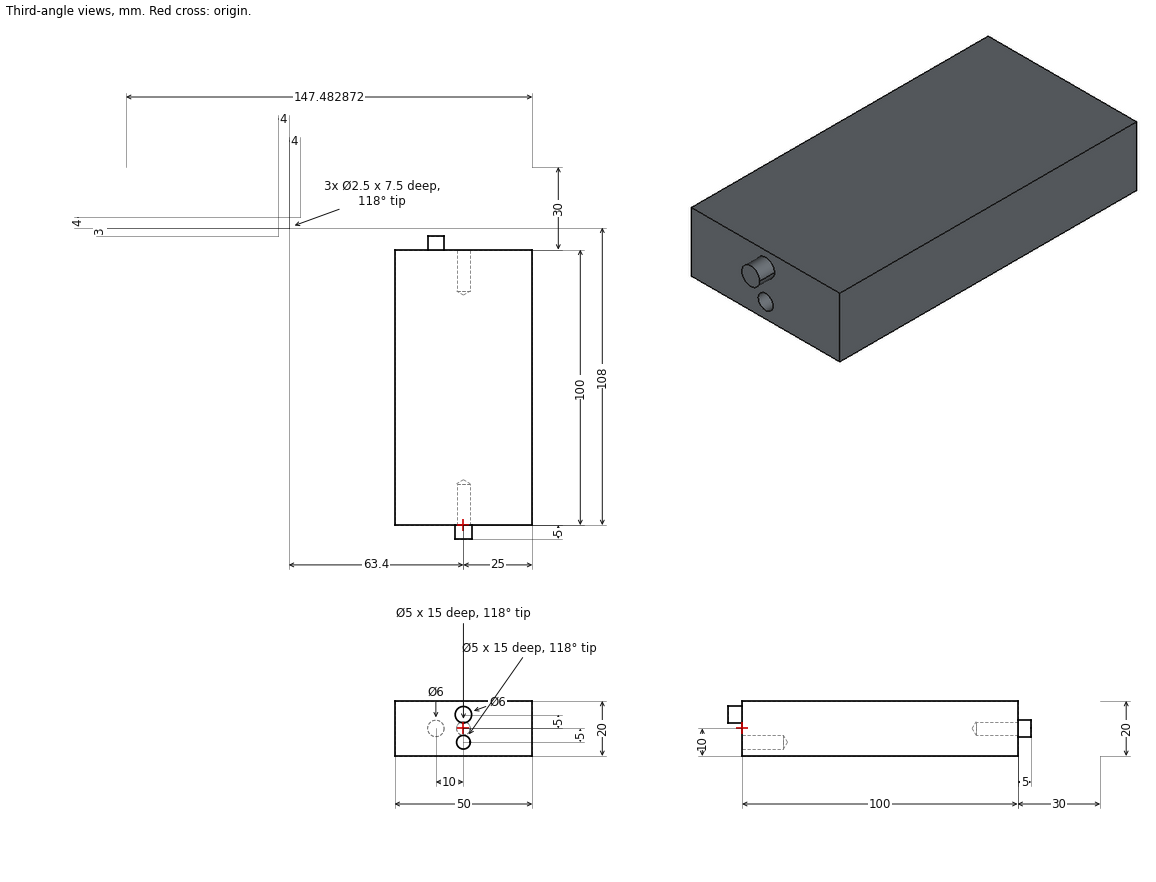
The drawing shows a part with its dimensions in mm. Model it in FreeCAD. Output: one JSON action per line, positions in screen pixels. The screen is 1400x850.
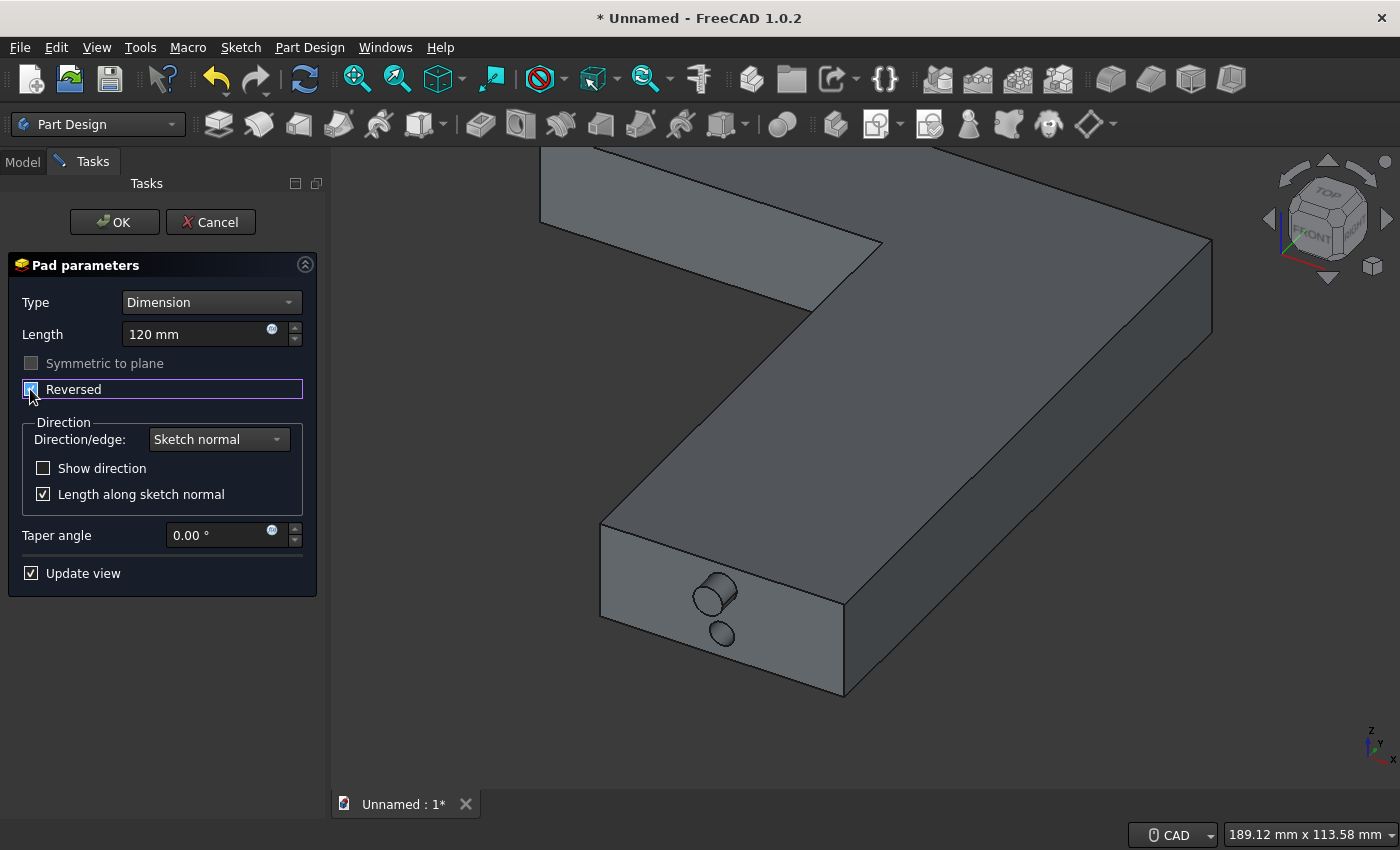
{"action": "left_click", "coordinate": [115, 222]}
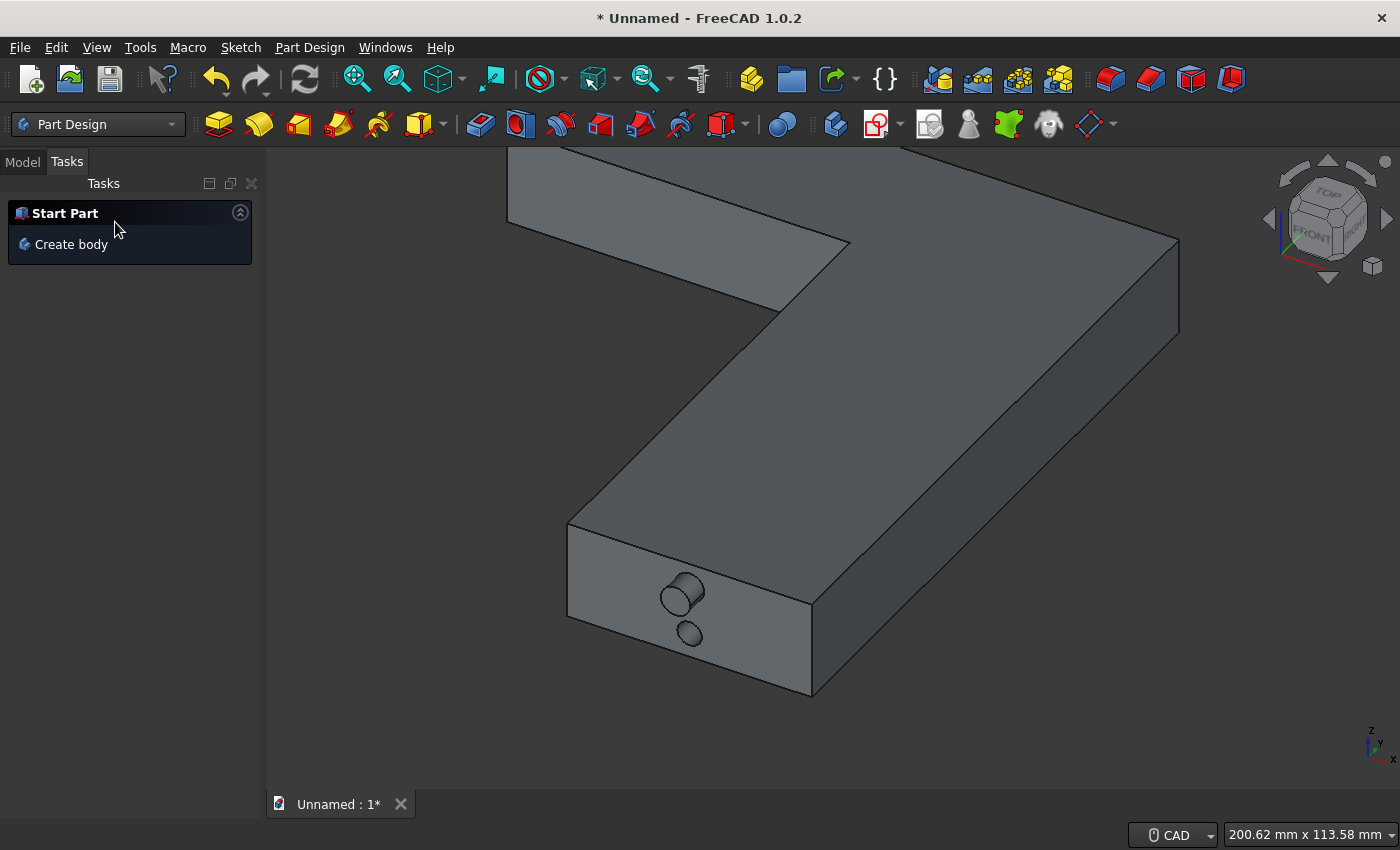
{"action": "left_click", "coordinate": [358, 80]}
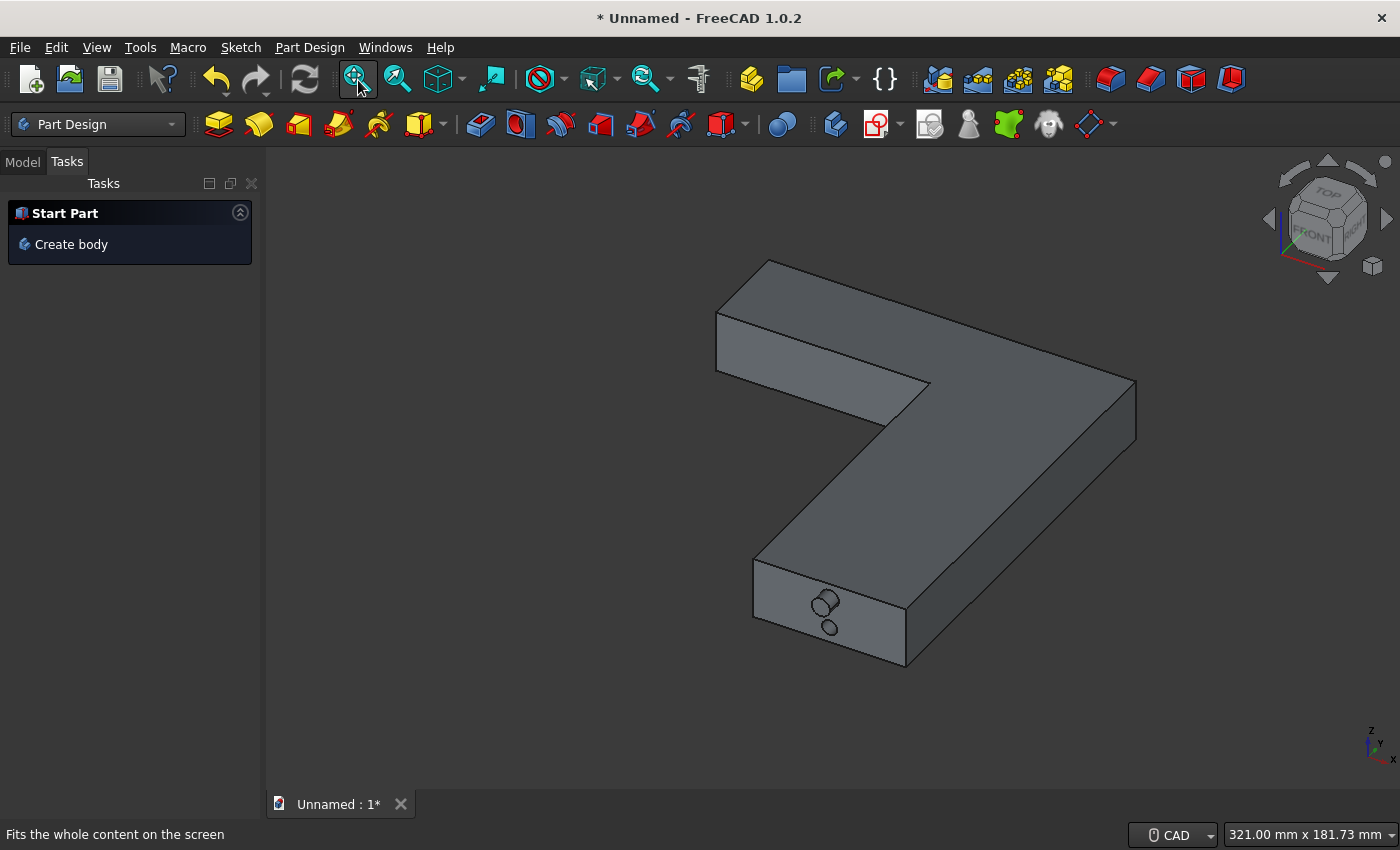
{"action": "left_click", "coordinate": [1008, 403]}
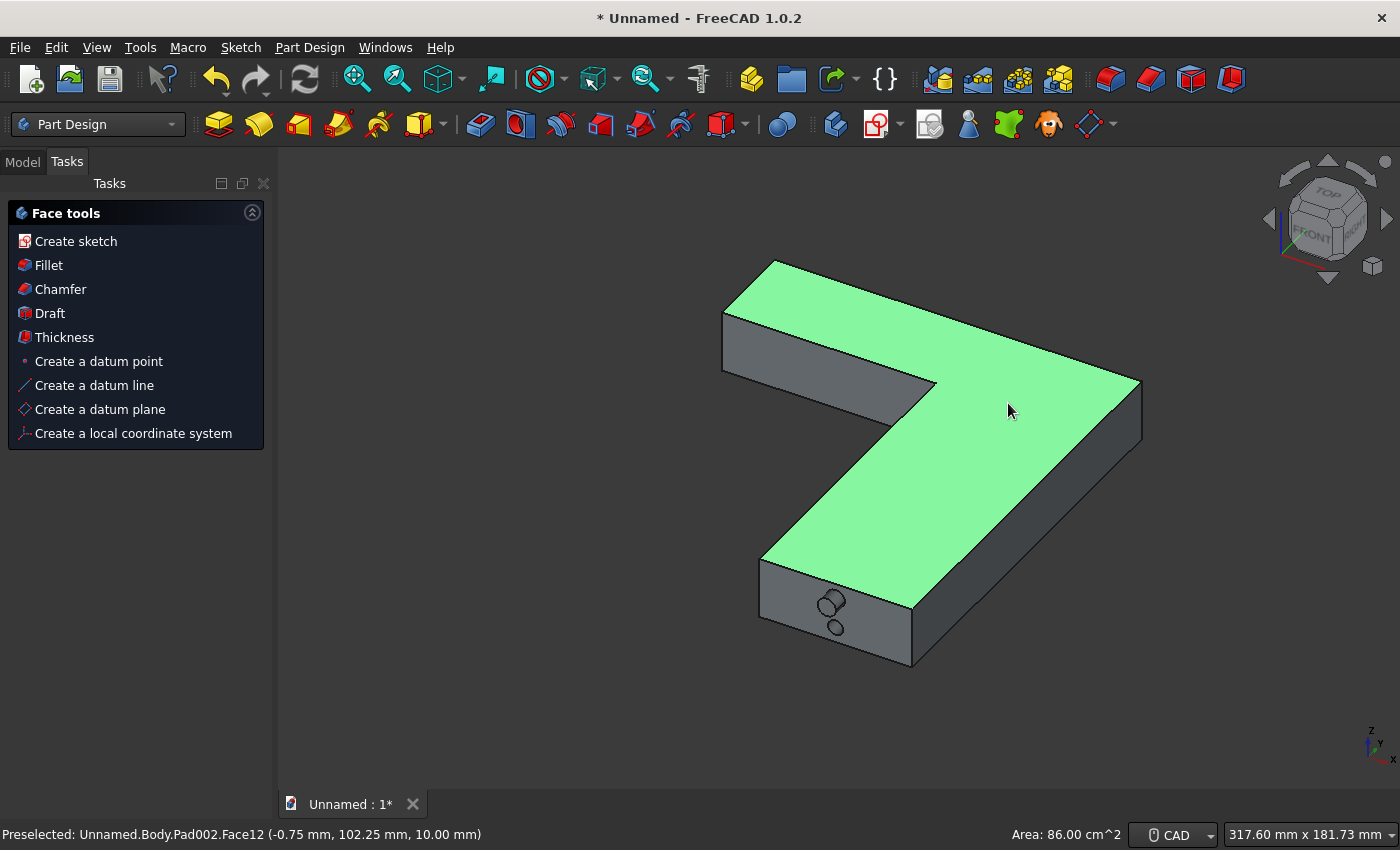
{"action": "left_click", "coordinate": [876, 124]}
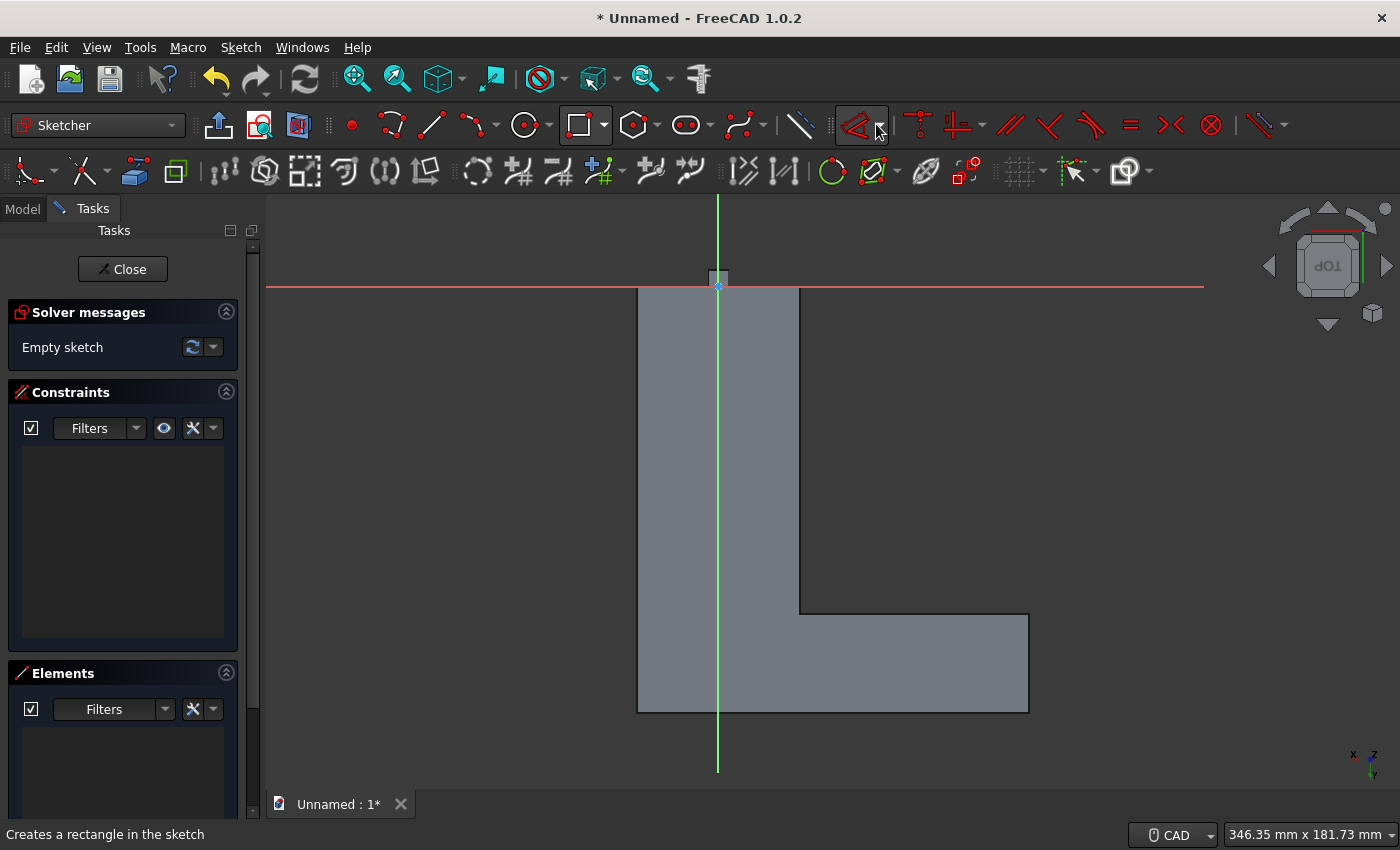
{"action": "scroll", "coordinate": [939, 654], "scroll_direction": "up", "scroll_amount": 13}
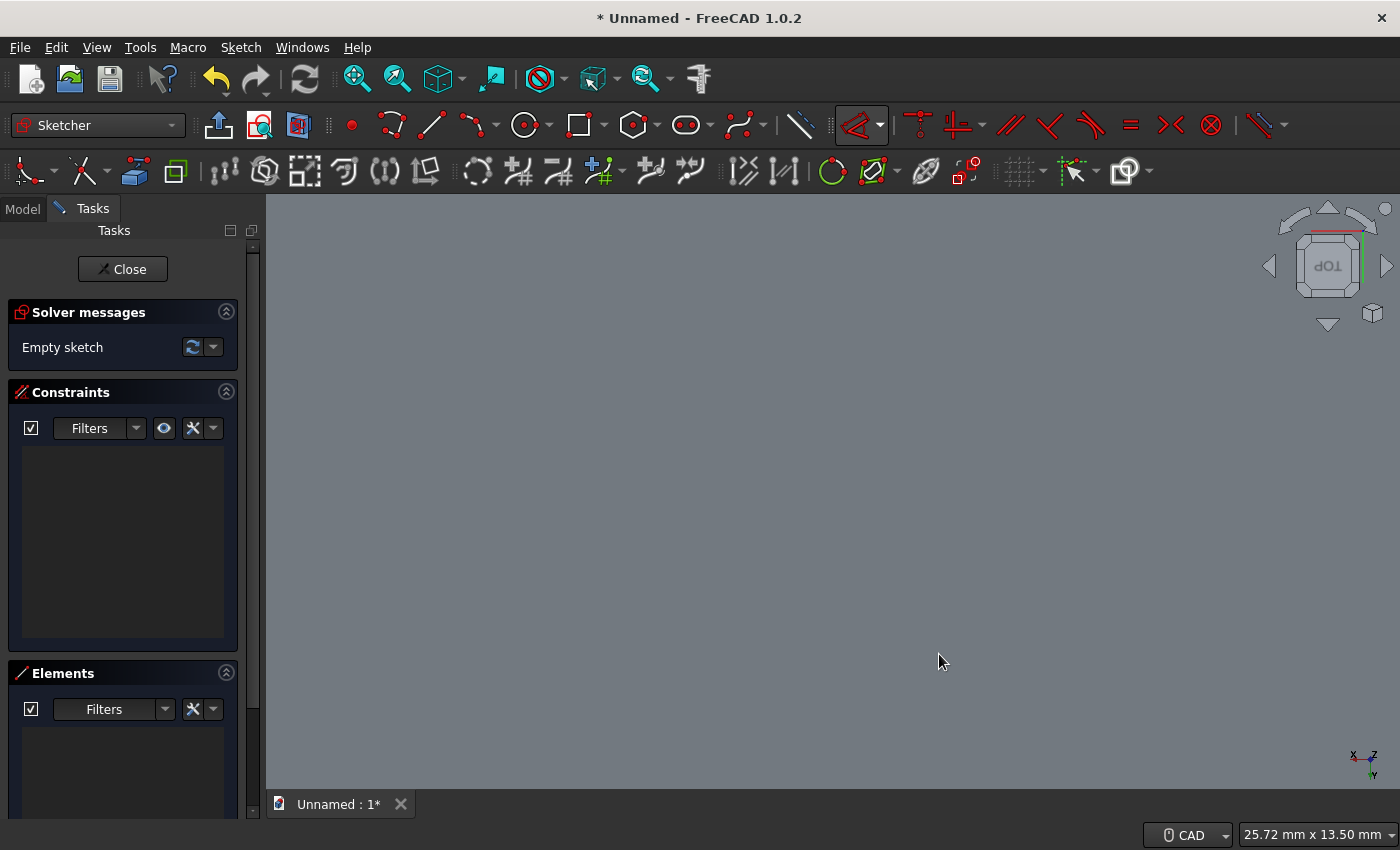
{"action": "key", "text": "g c"}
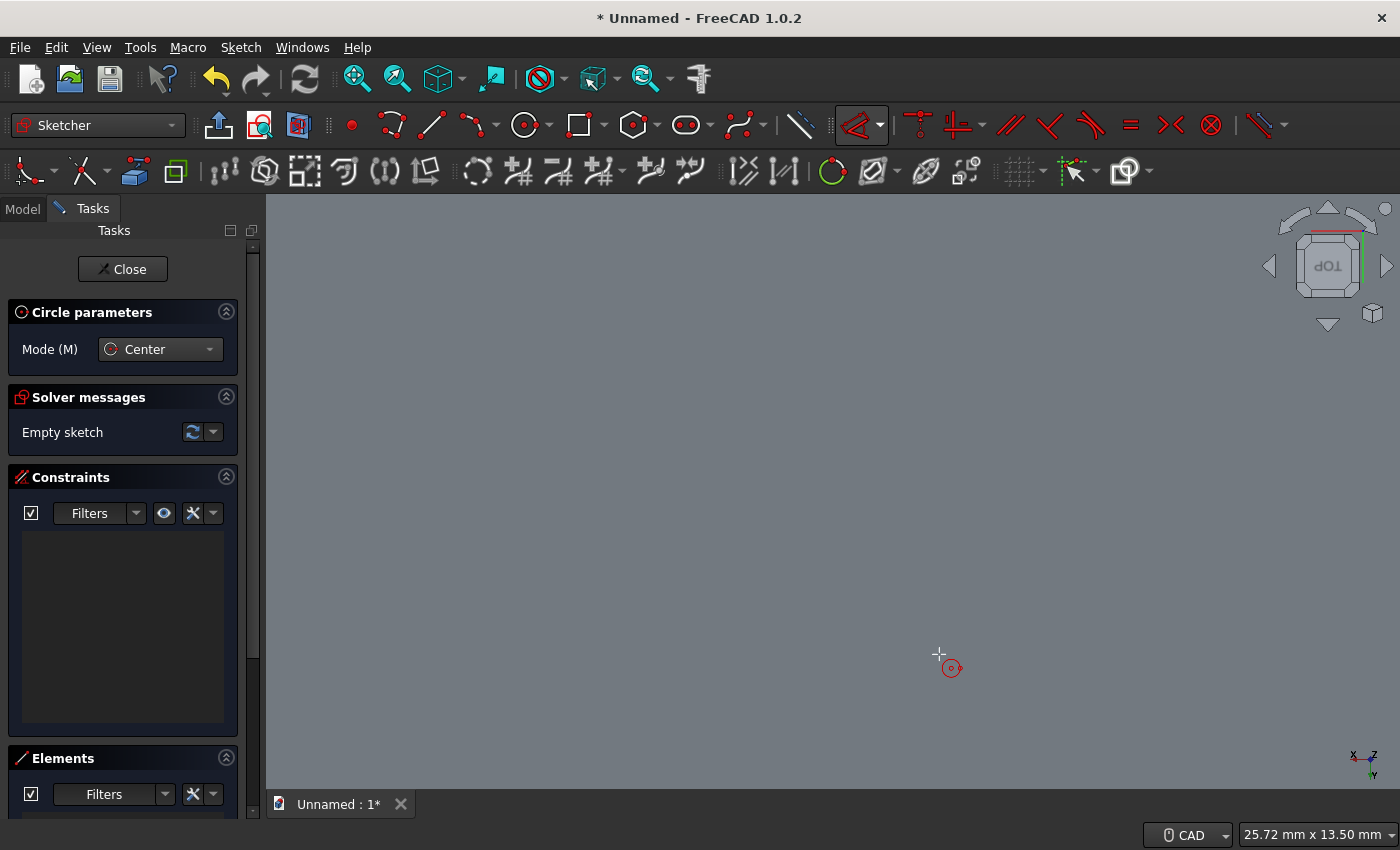
{"action": "left_click", "coordinate": [756, 462]}
{"action": "left_click", "coordinate": [795, 423]}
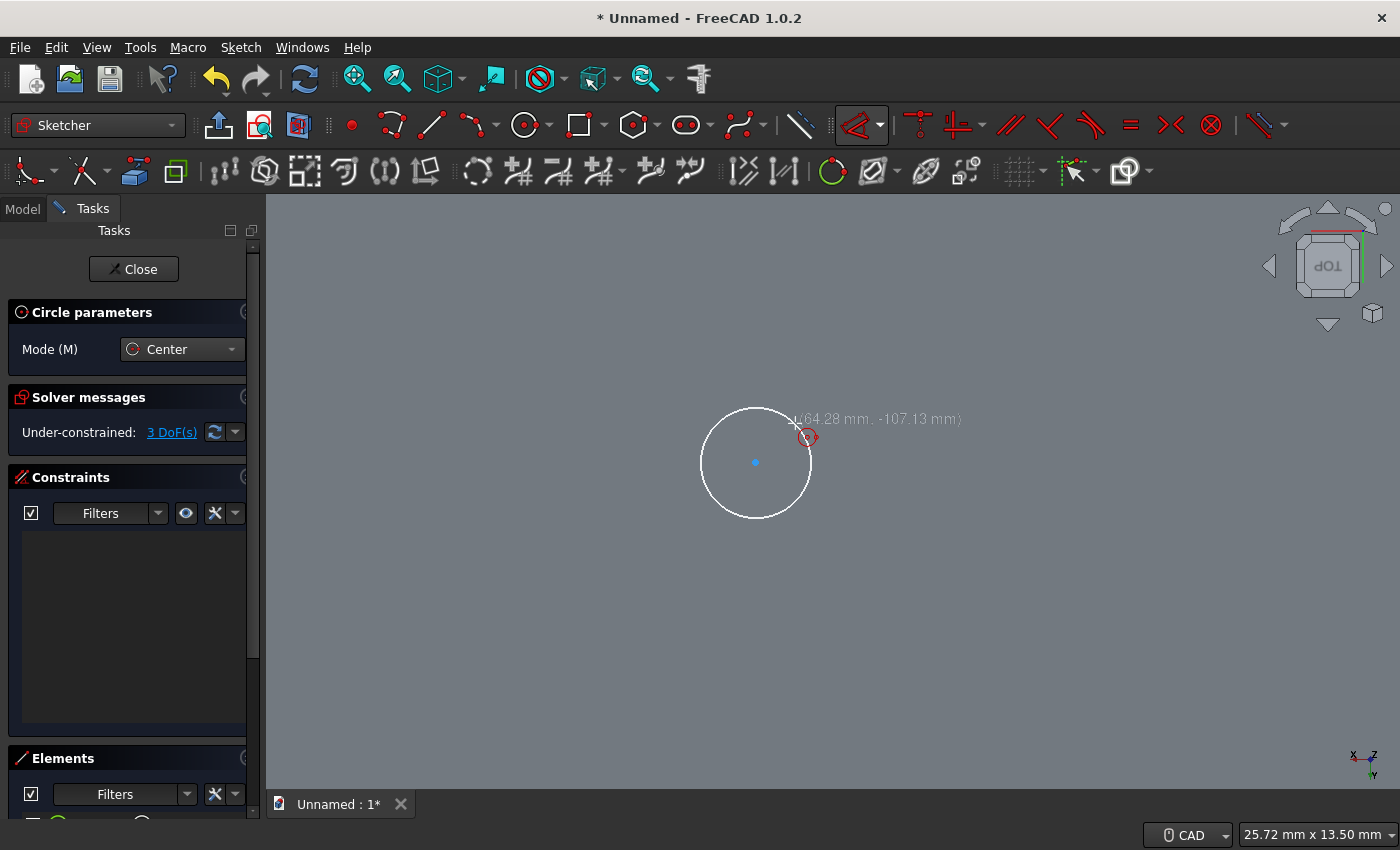
{"action": "left_click", "coordinate": [580, 639]}
{"action": "left_click", "coordinate": [619, 600]}